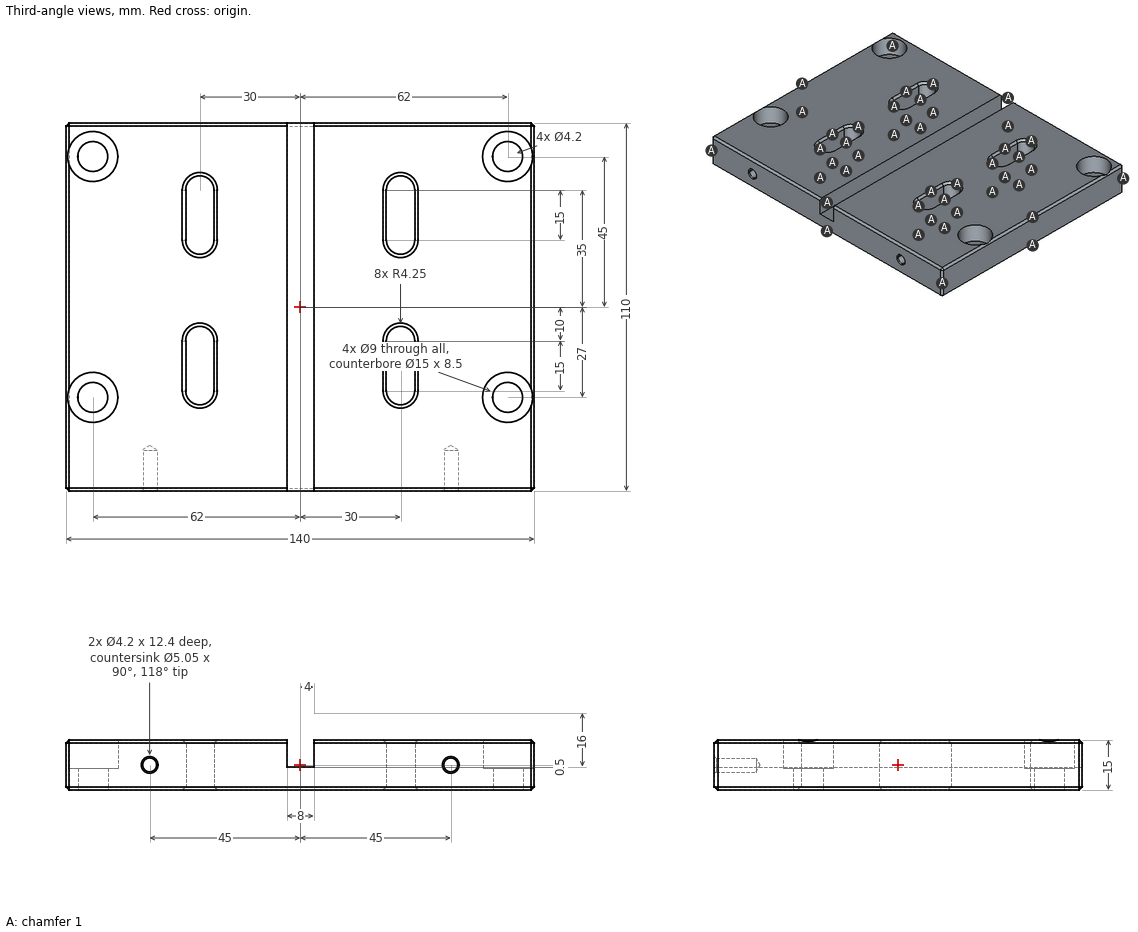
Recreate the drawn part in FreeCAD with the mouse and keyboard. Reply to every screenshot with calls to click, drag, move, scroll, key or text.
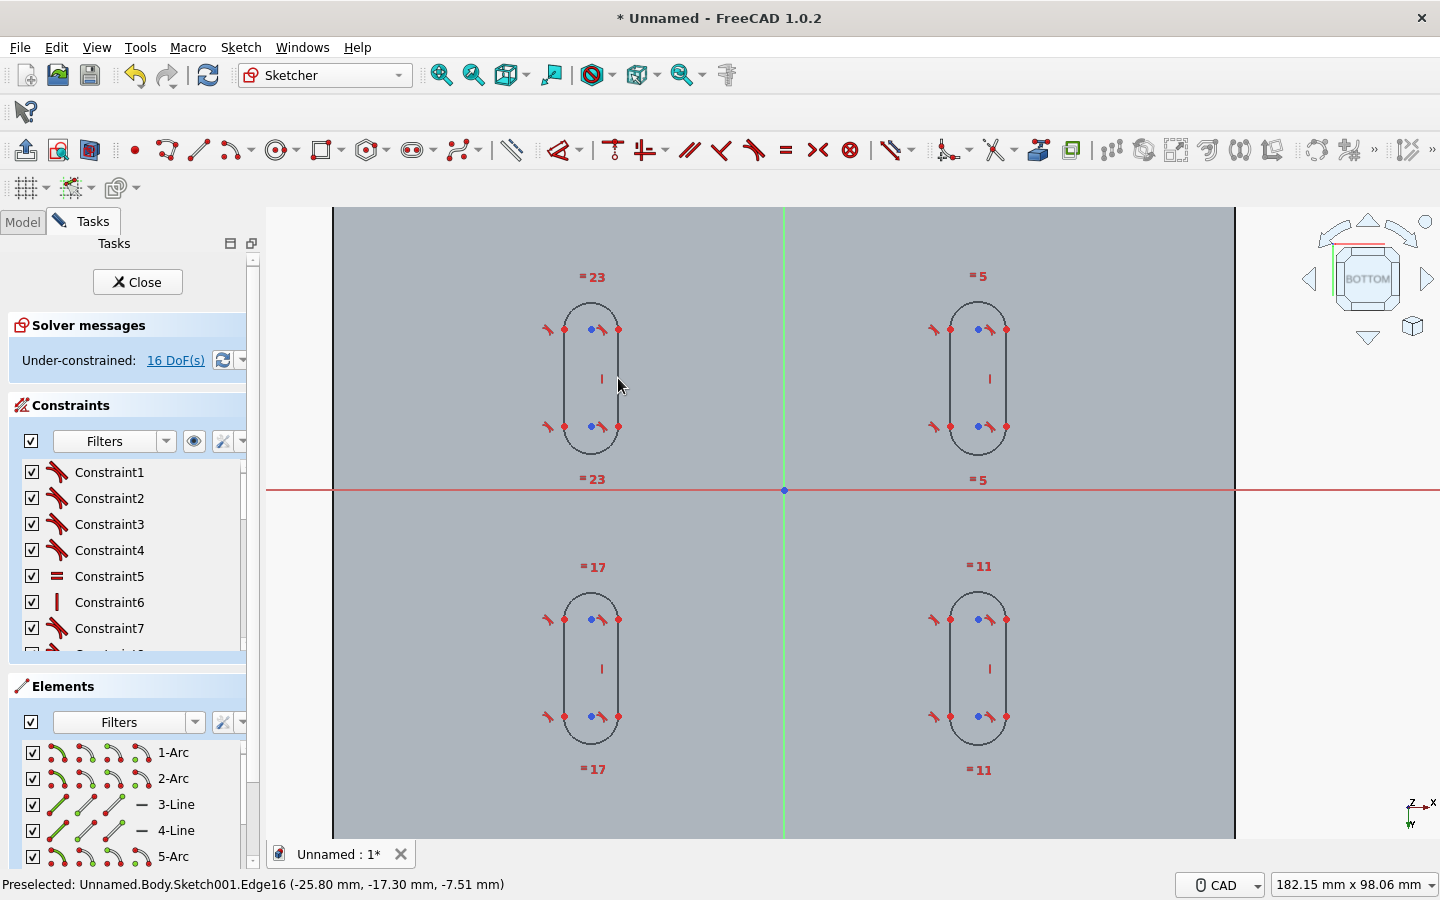
click(962, 450)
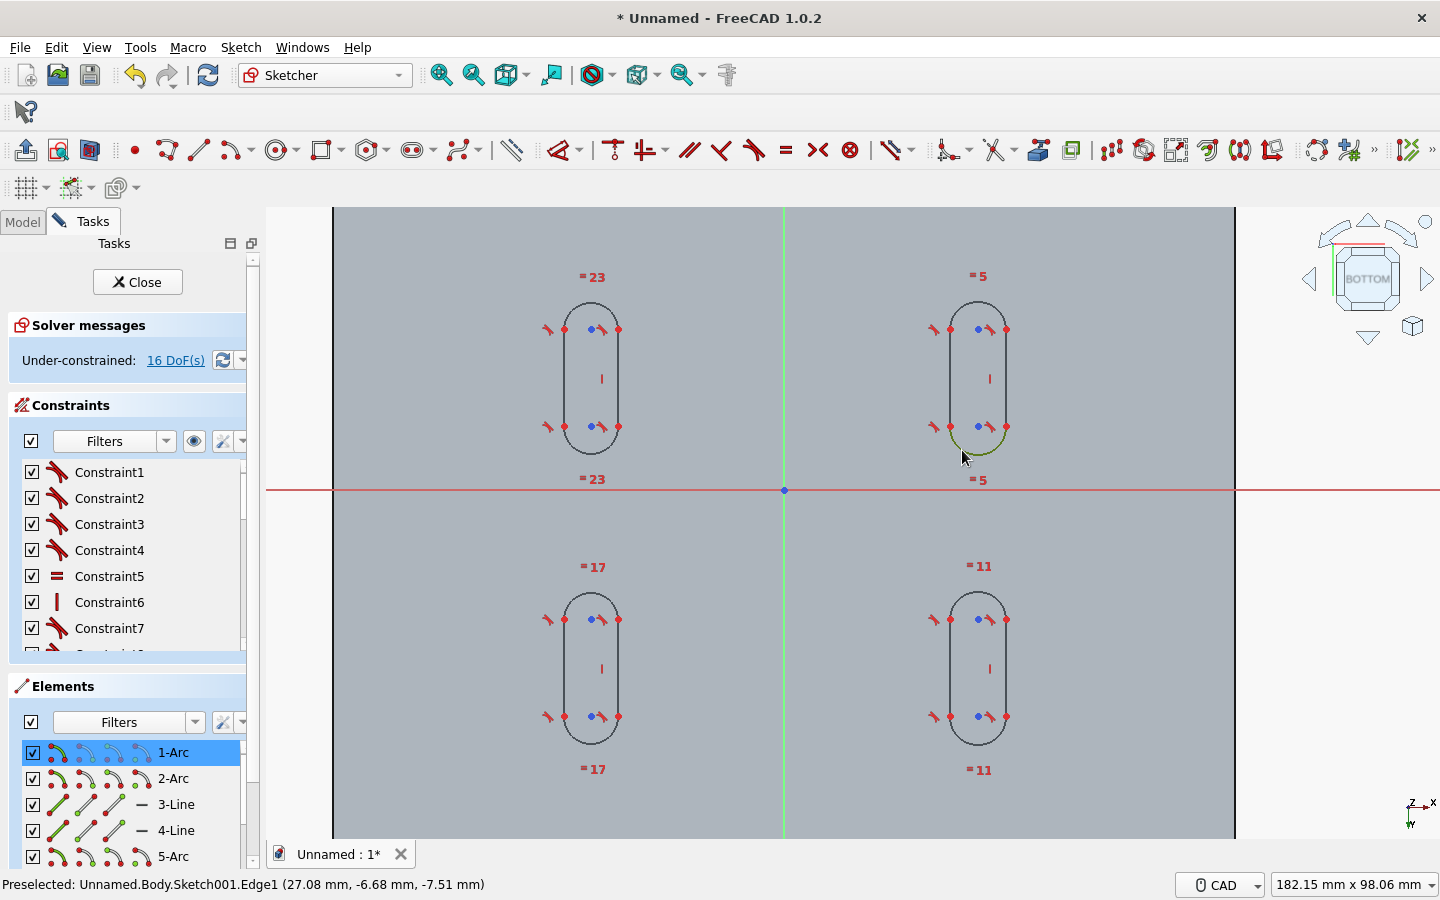
click(962, 740)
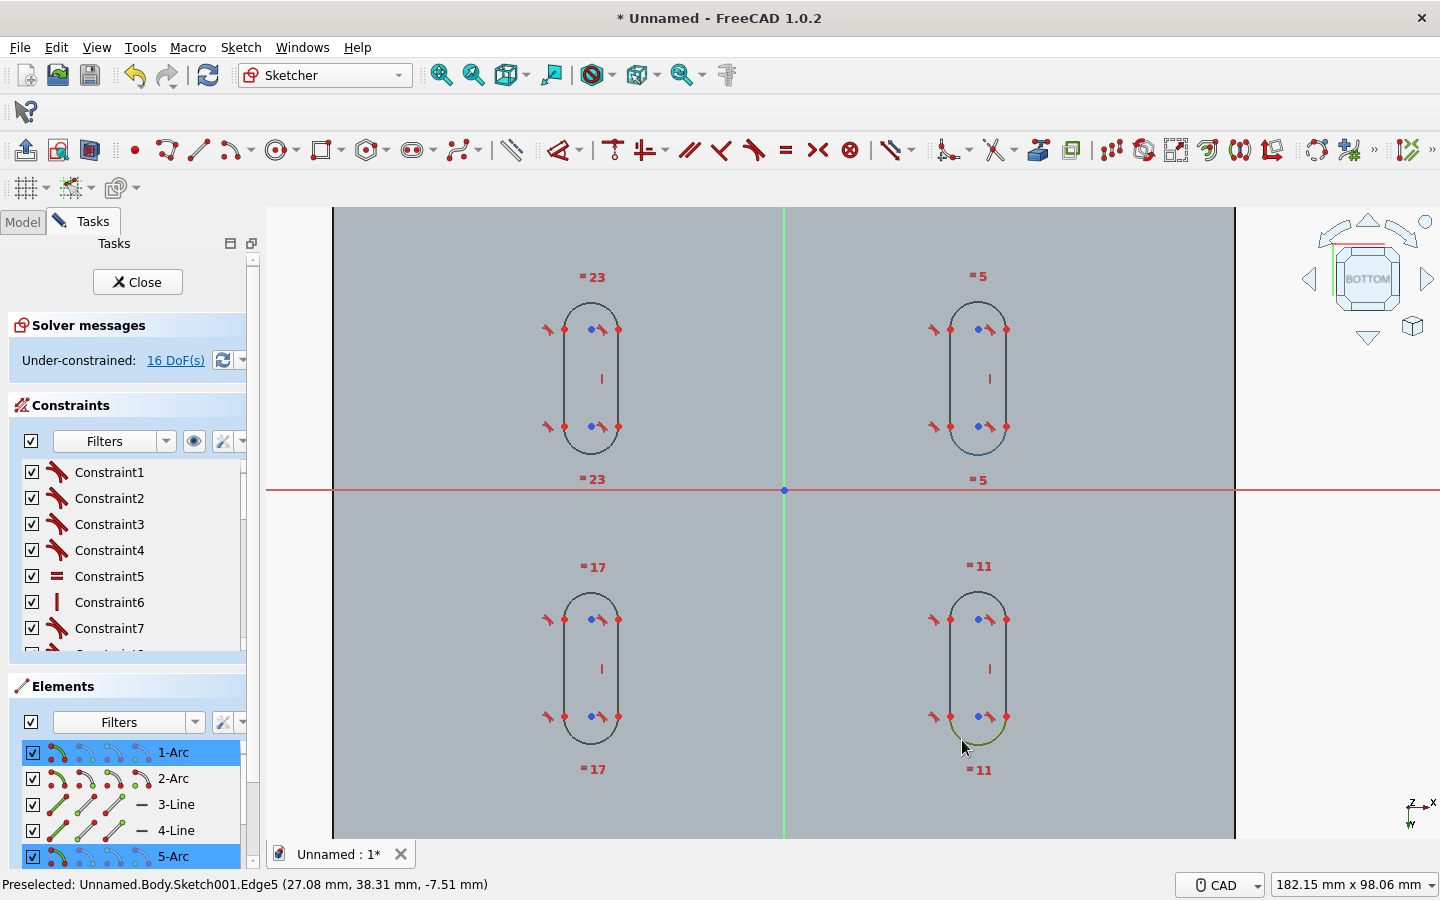
click(575, 739)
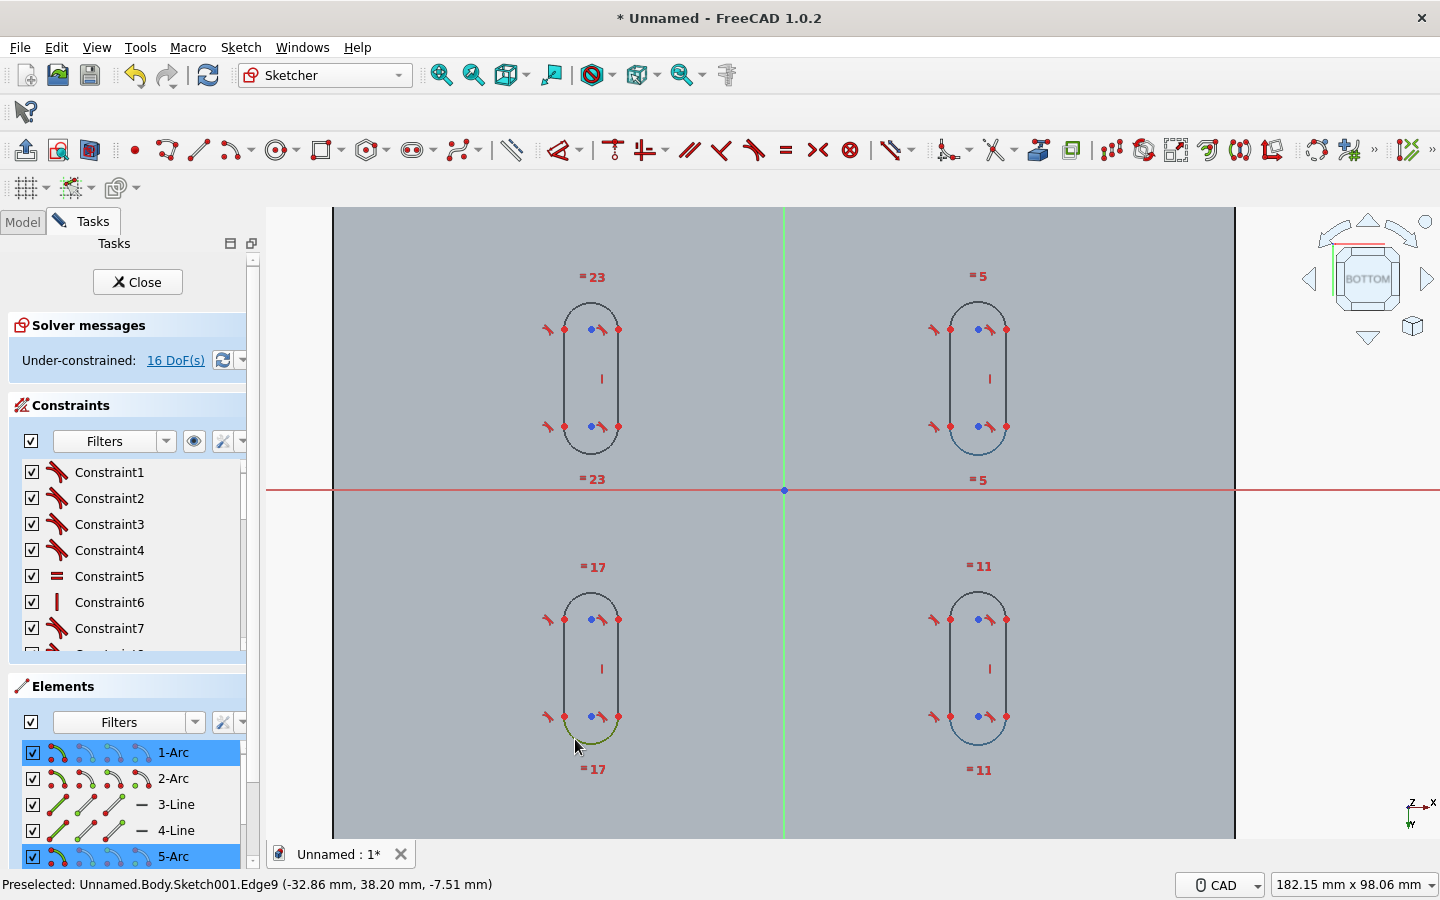
click(575, 449)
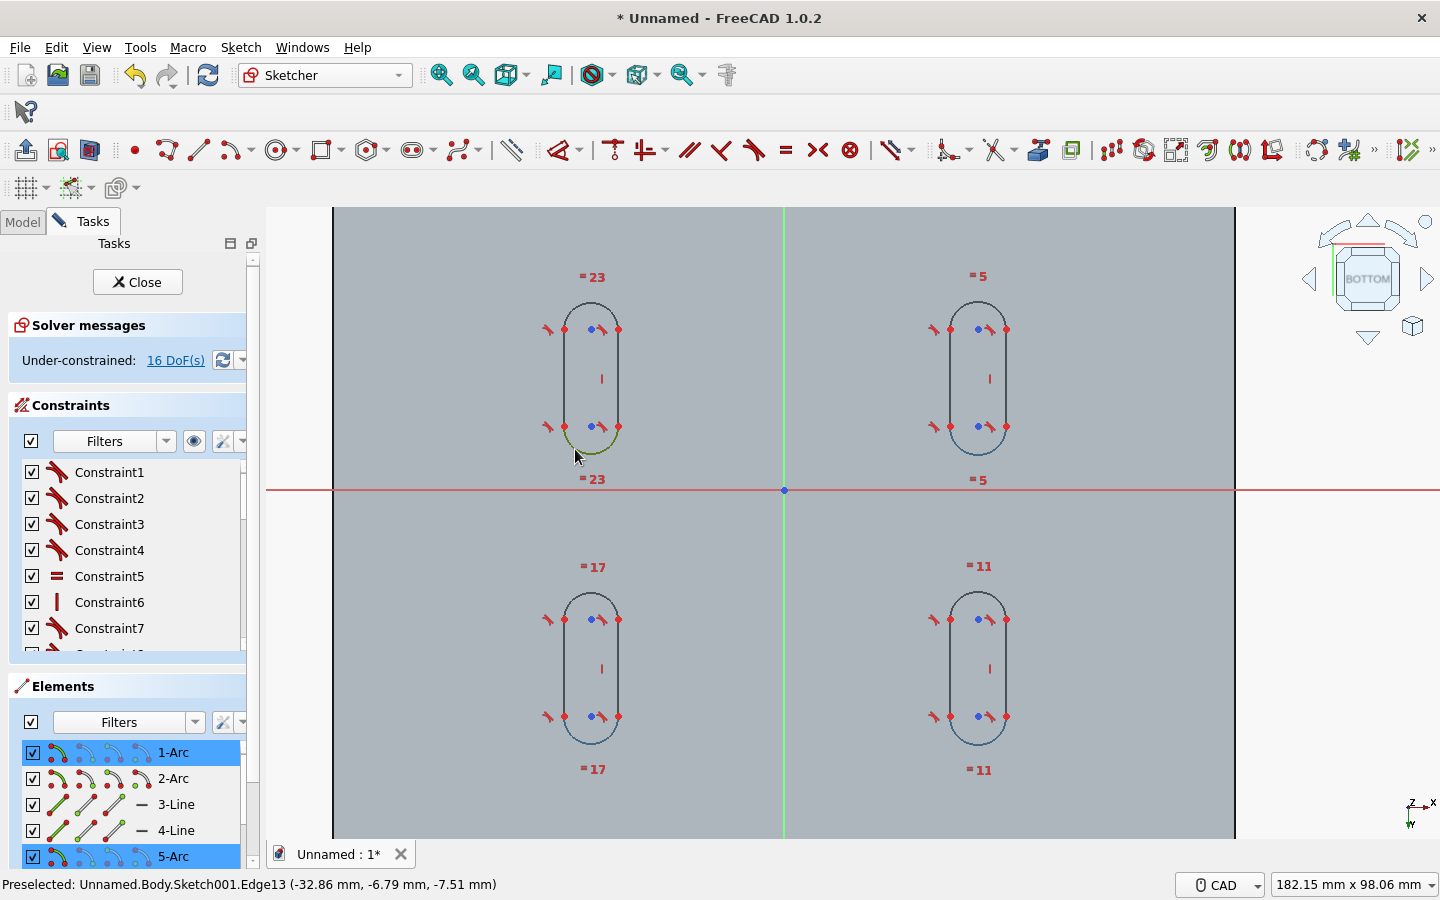
key(e)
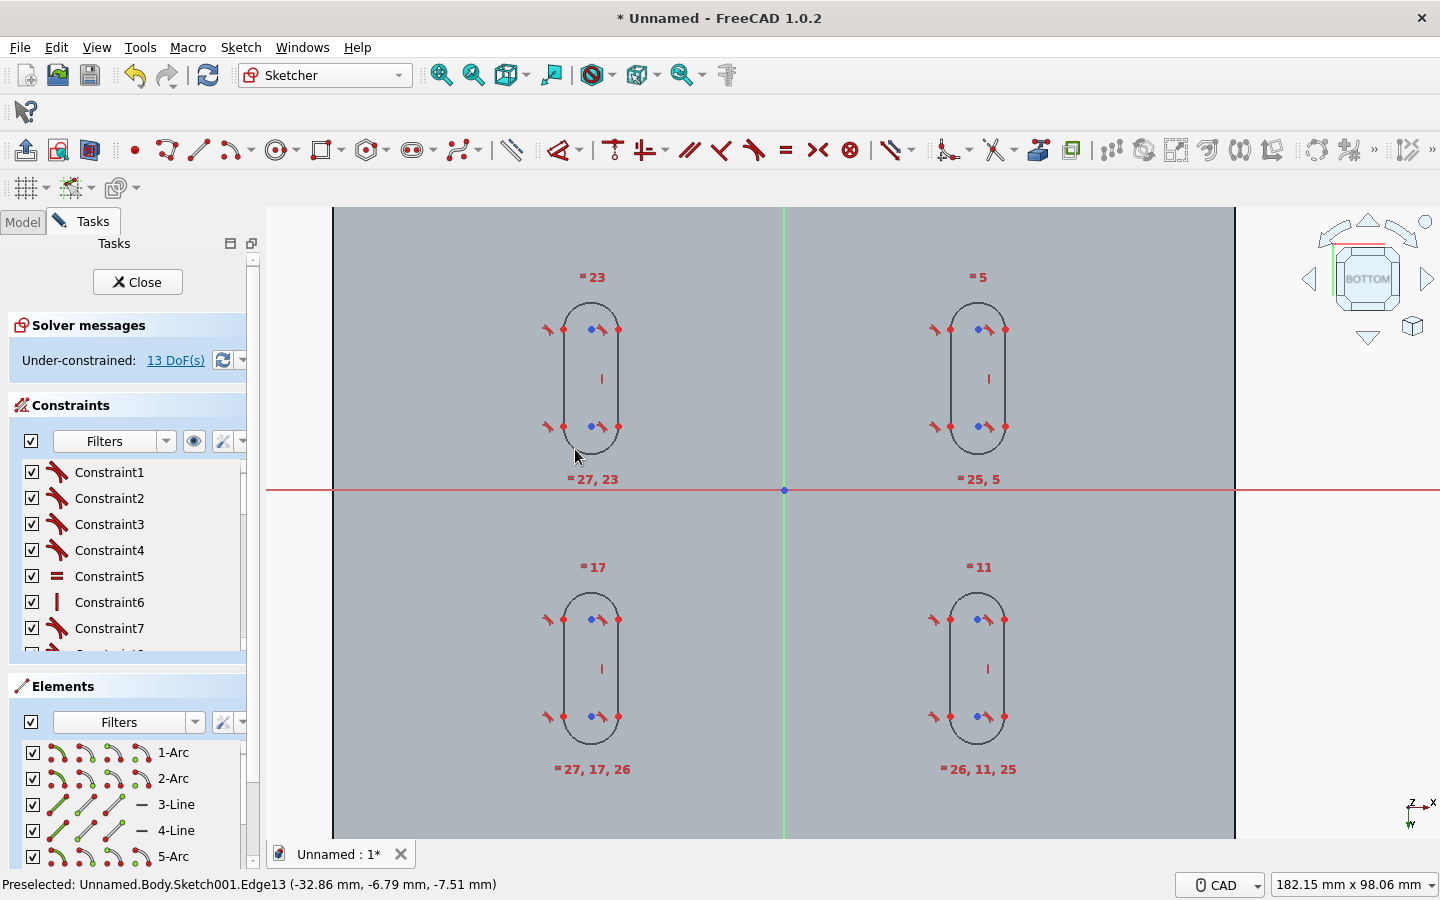
key(d)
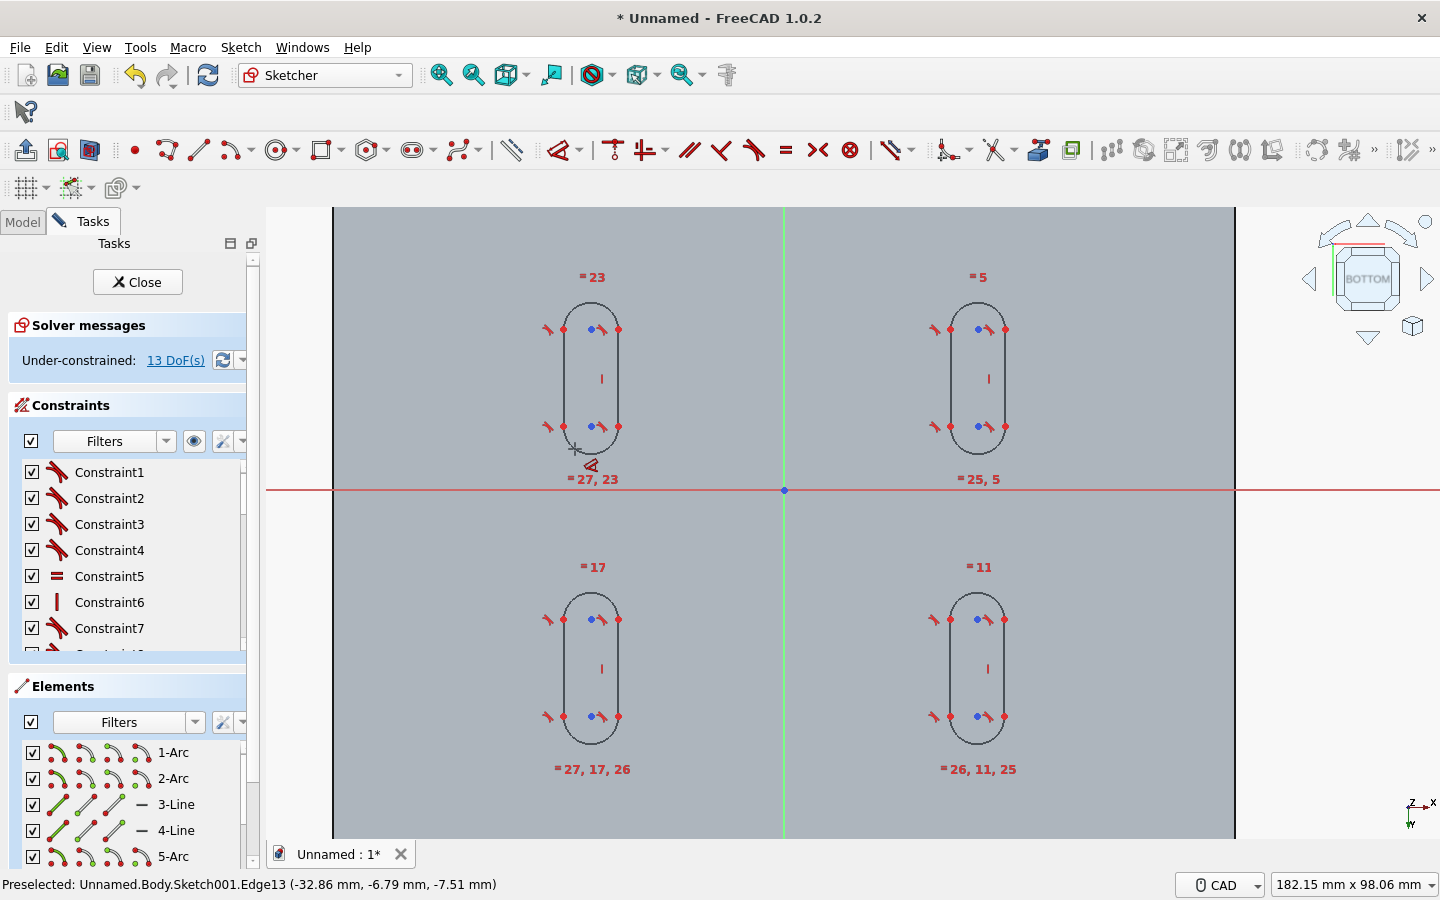
scroll(962, 449, up, 2)